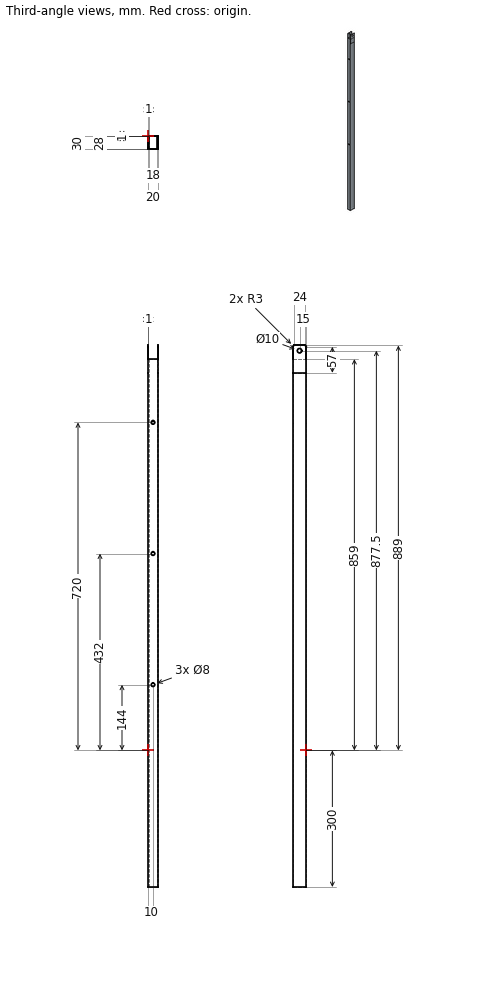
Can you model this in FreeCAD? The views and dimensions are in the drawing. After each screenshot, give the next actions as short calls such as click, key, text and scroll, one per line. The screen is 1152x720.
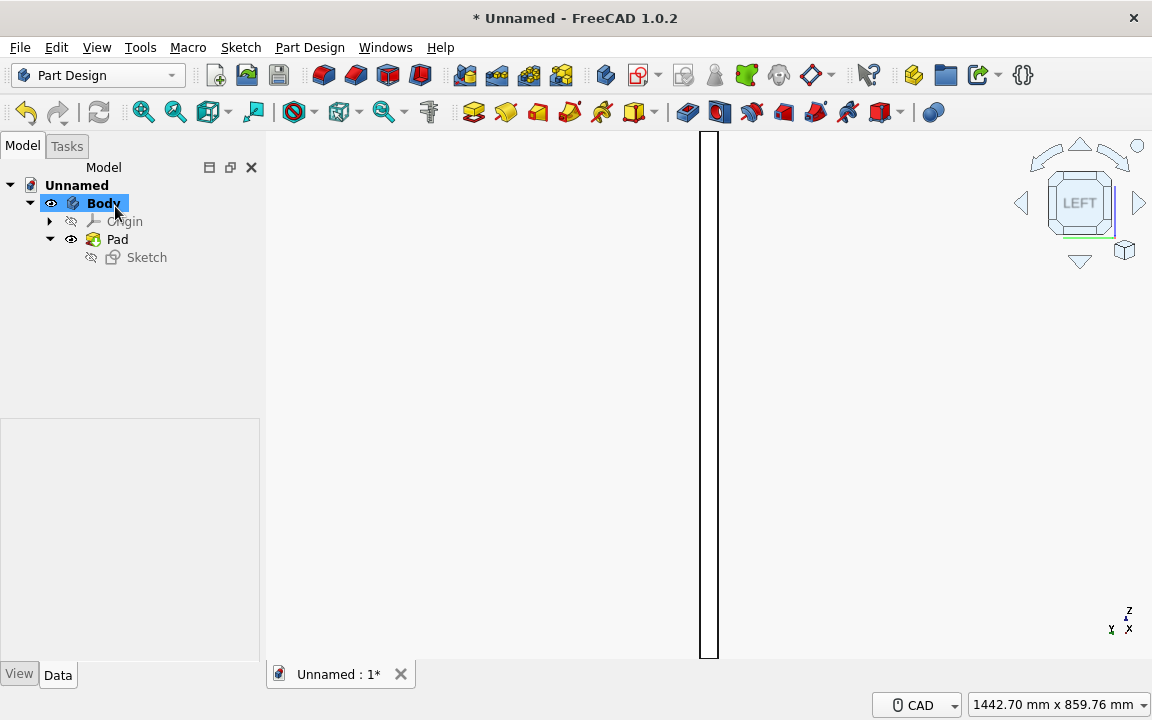
key(v)
key(f)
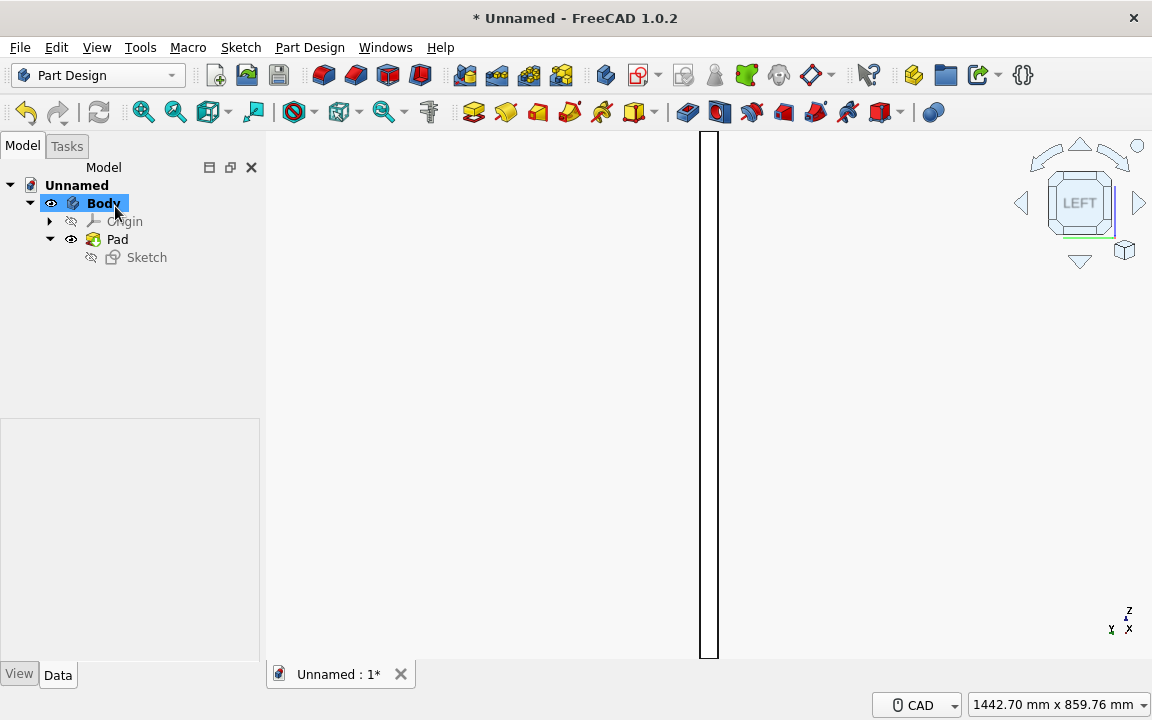
click(709, 168)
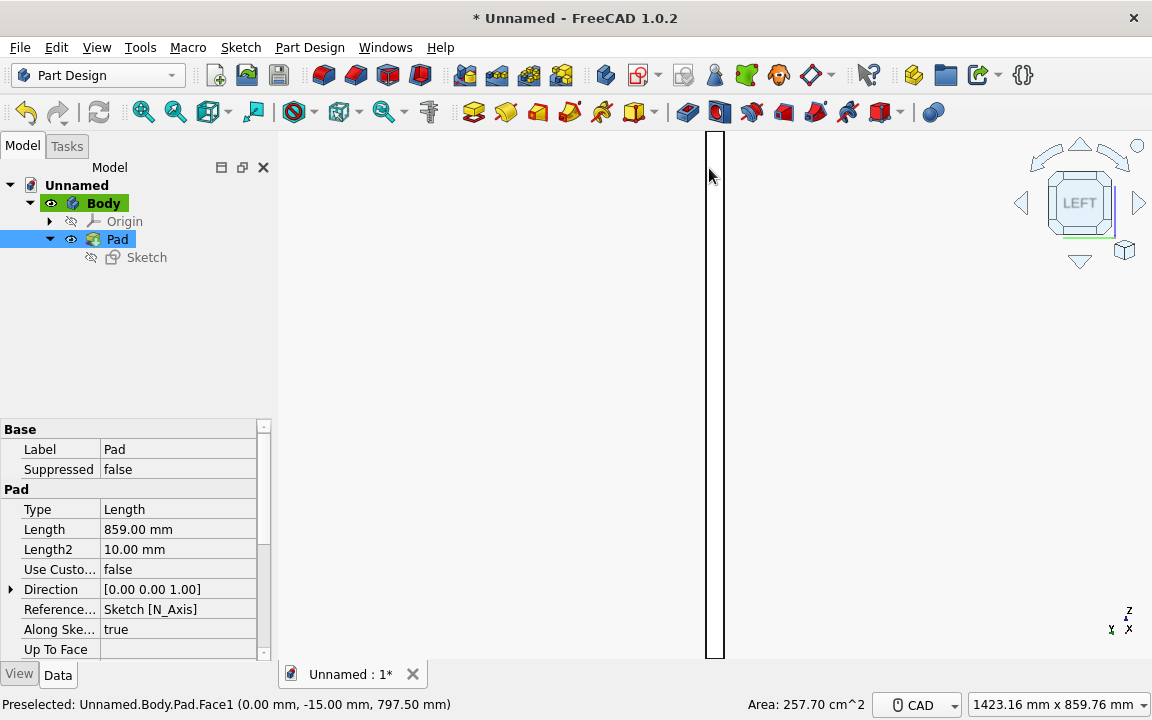
click(638, 76)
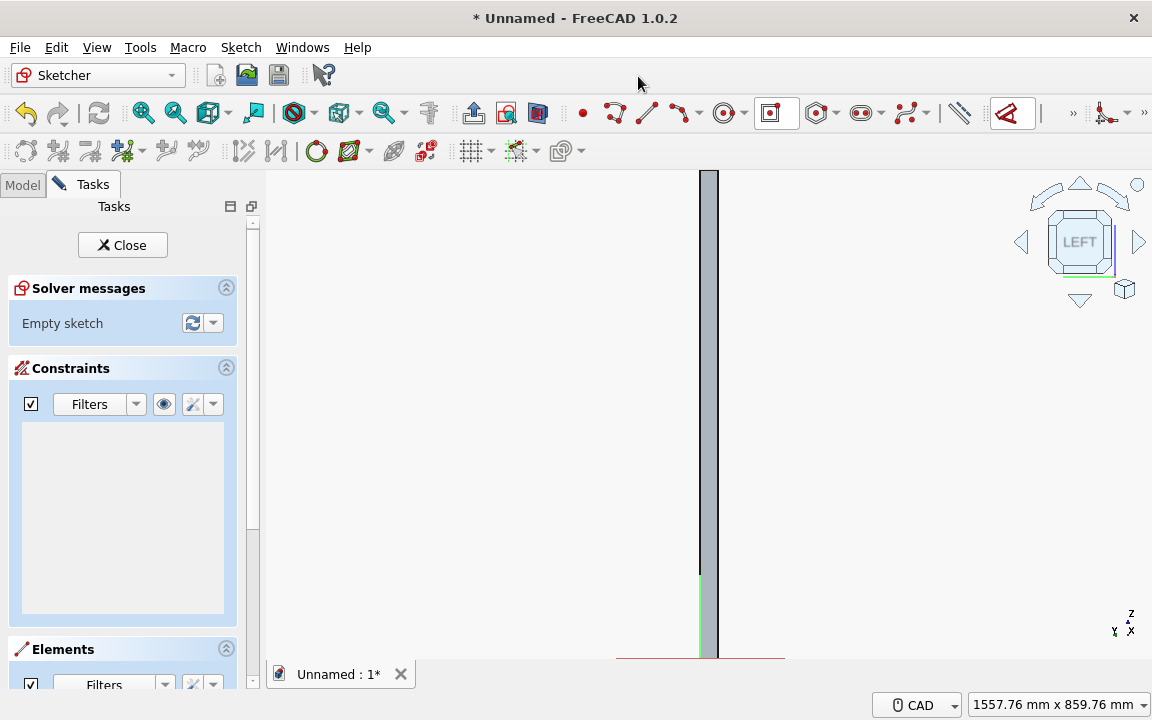
scroll(640, 414, down, 5)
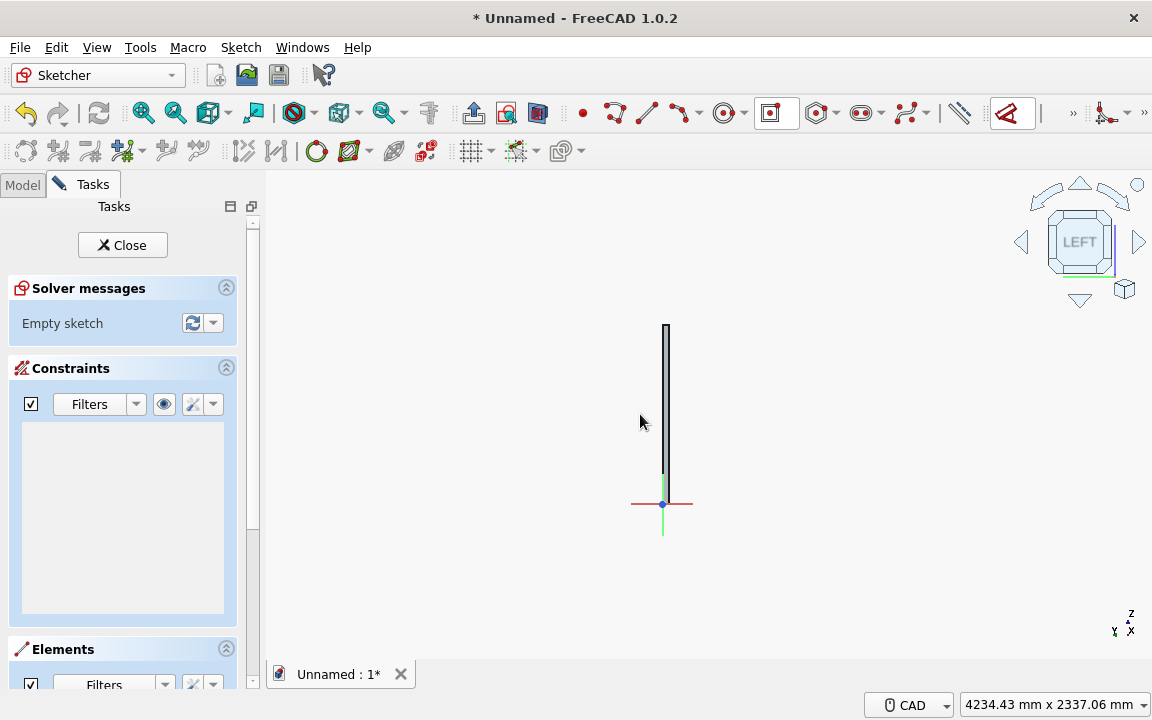
scroll(667, 320, up, 15)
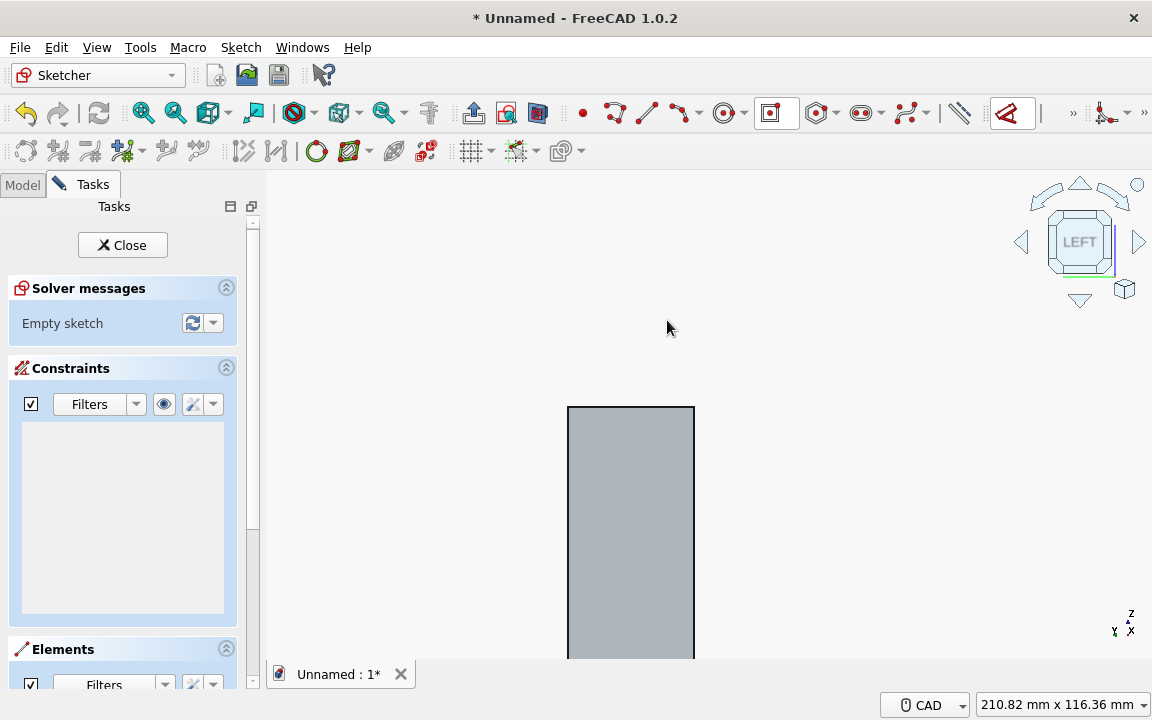
key(g)
key(l)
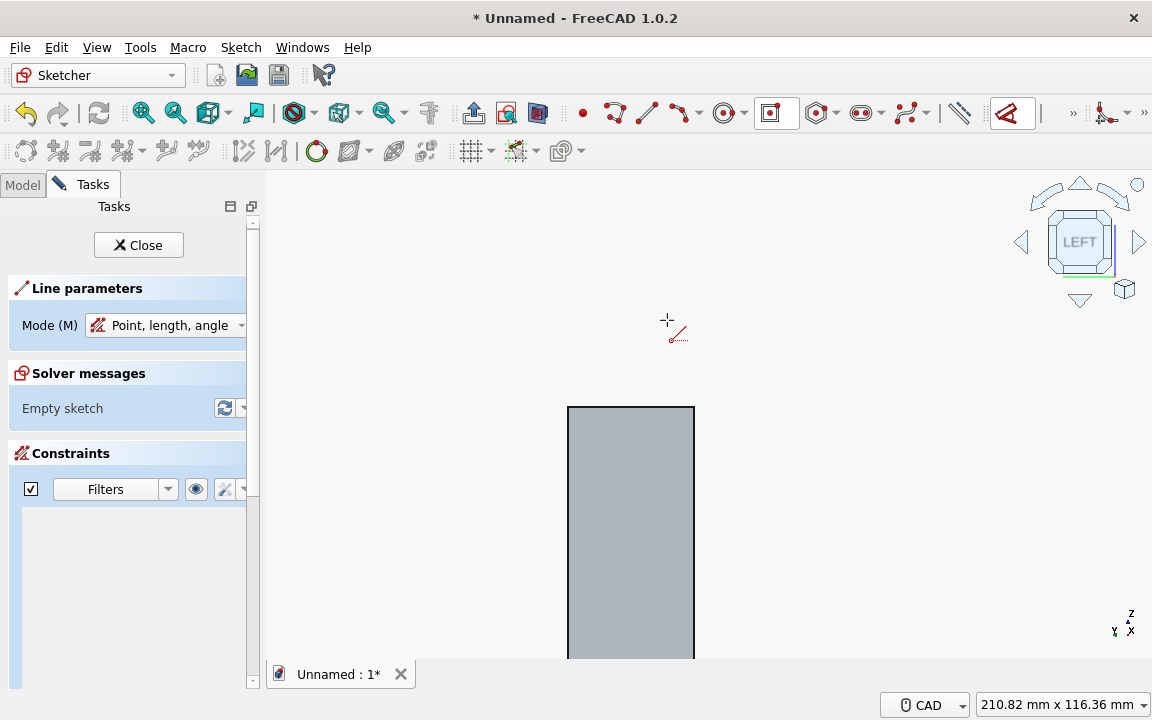
click(682, 281)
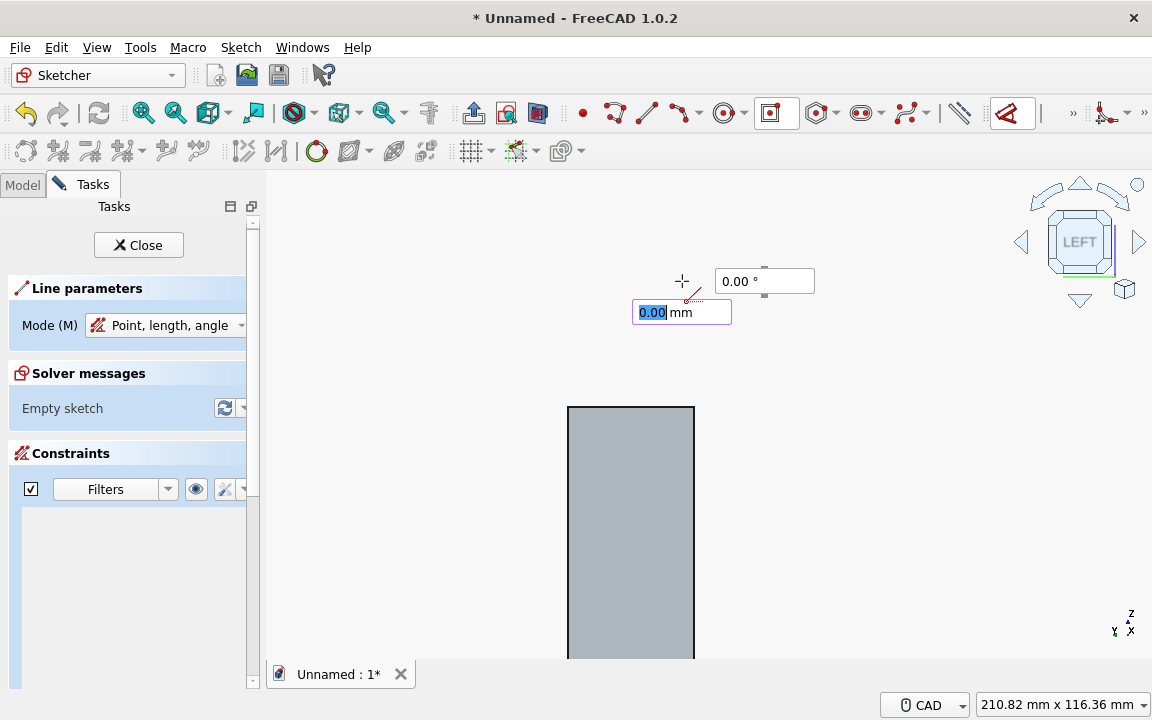
scroll(581, 281, up, 2)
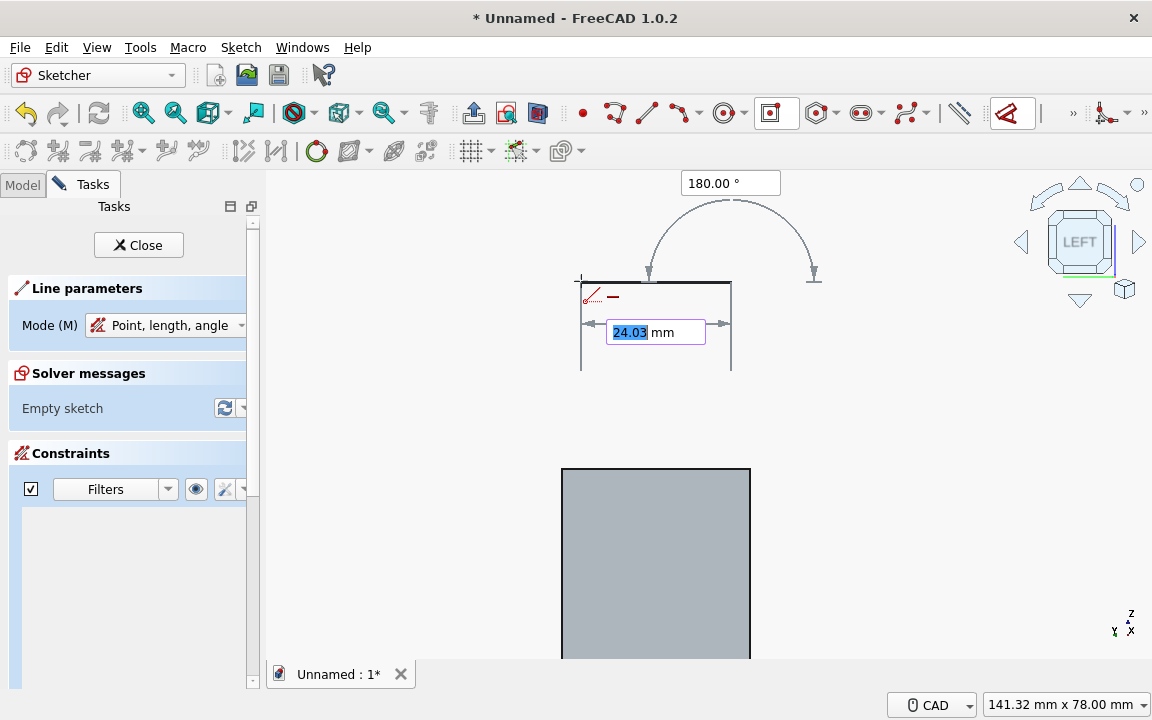
click(581, 281)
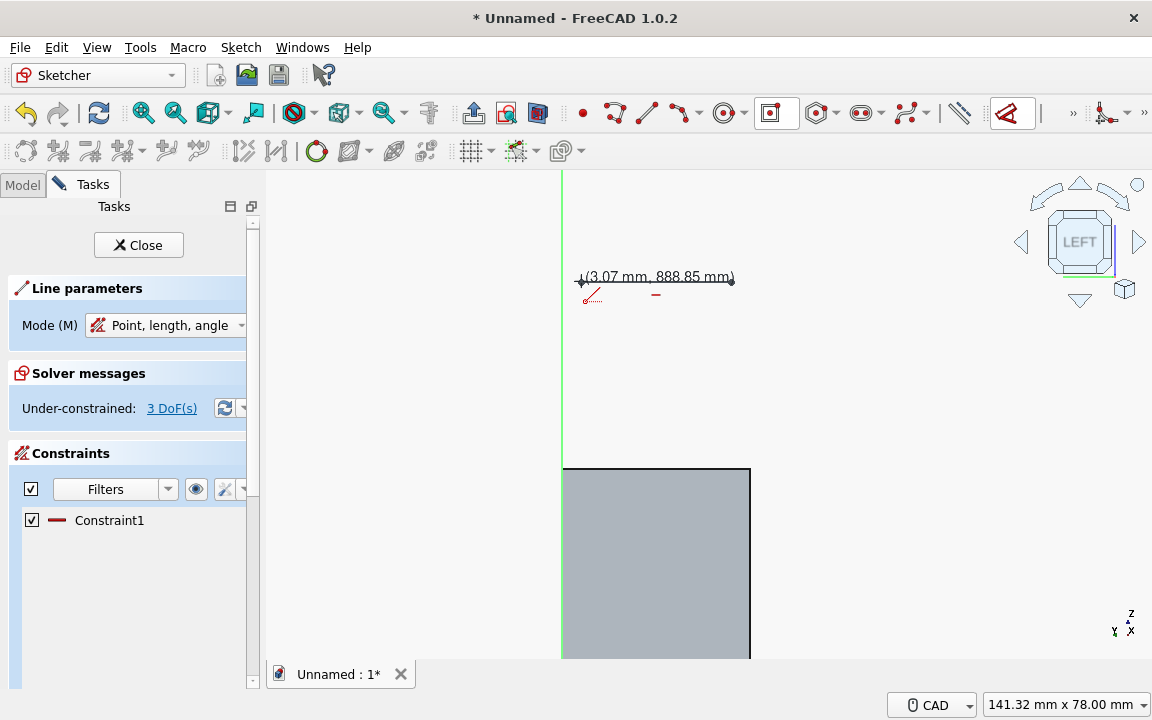
key(g)
key(m)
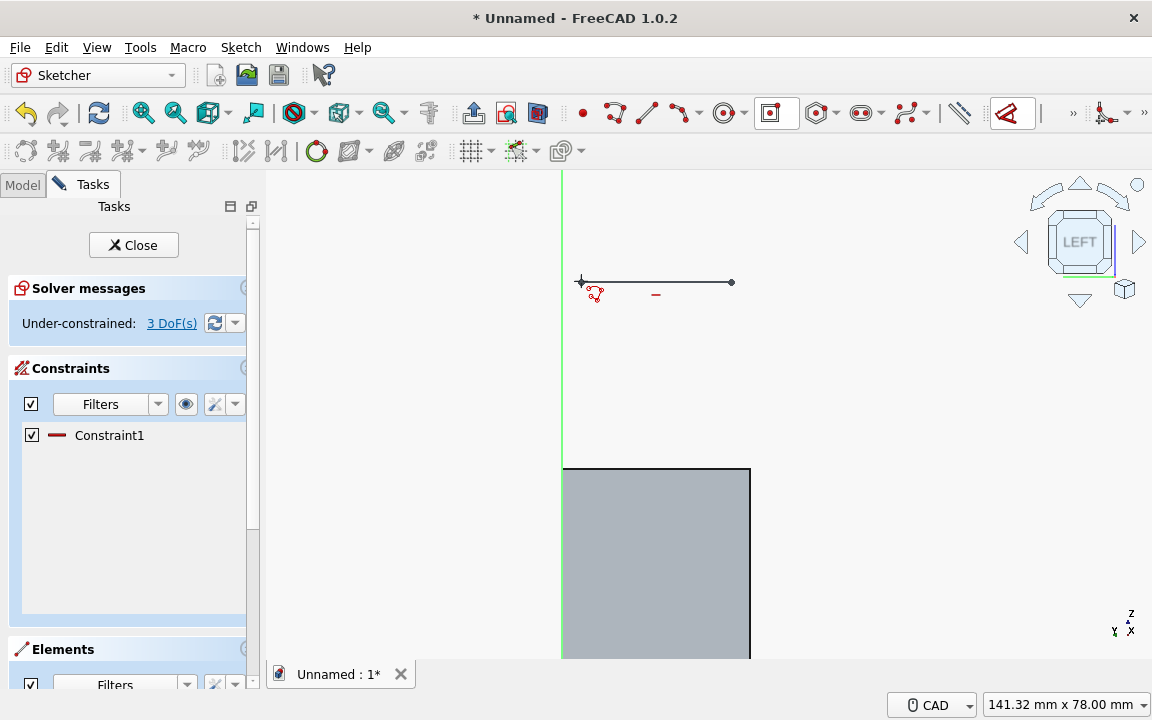
click(562, 300)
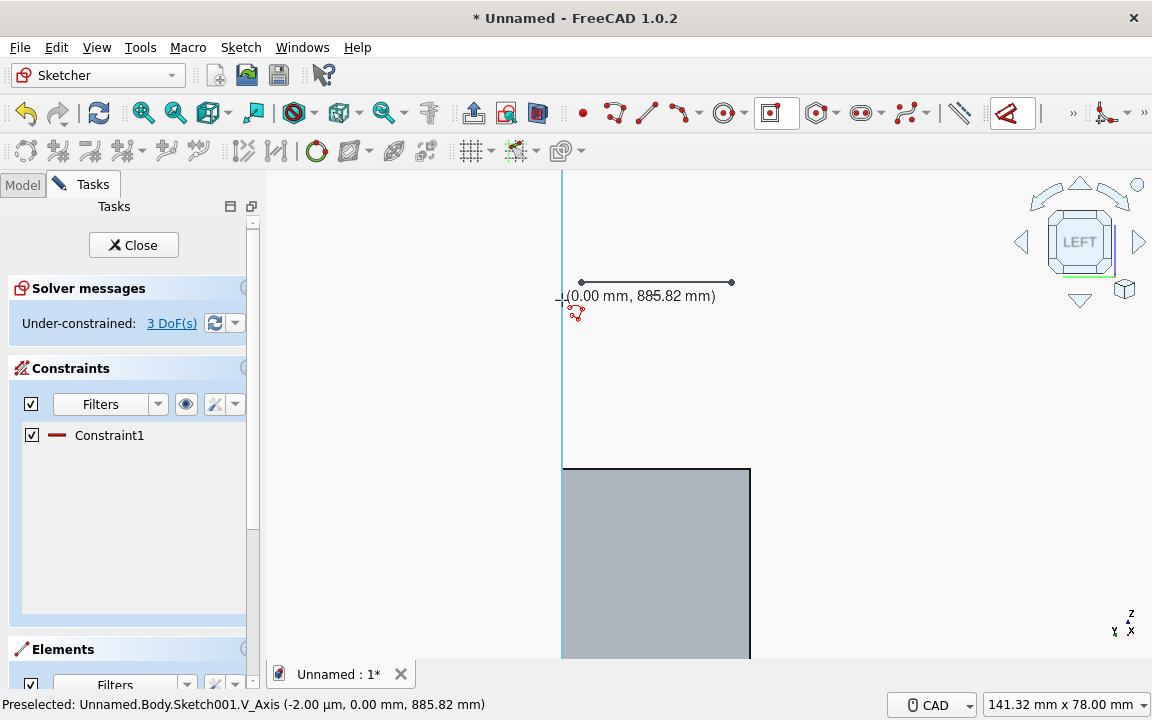
scroll(571, 198, down, 1)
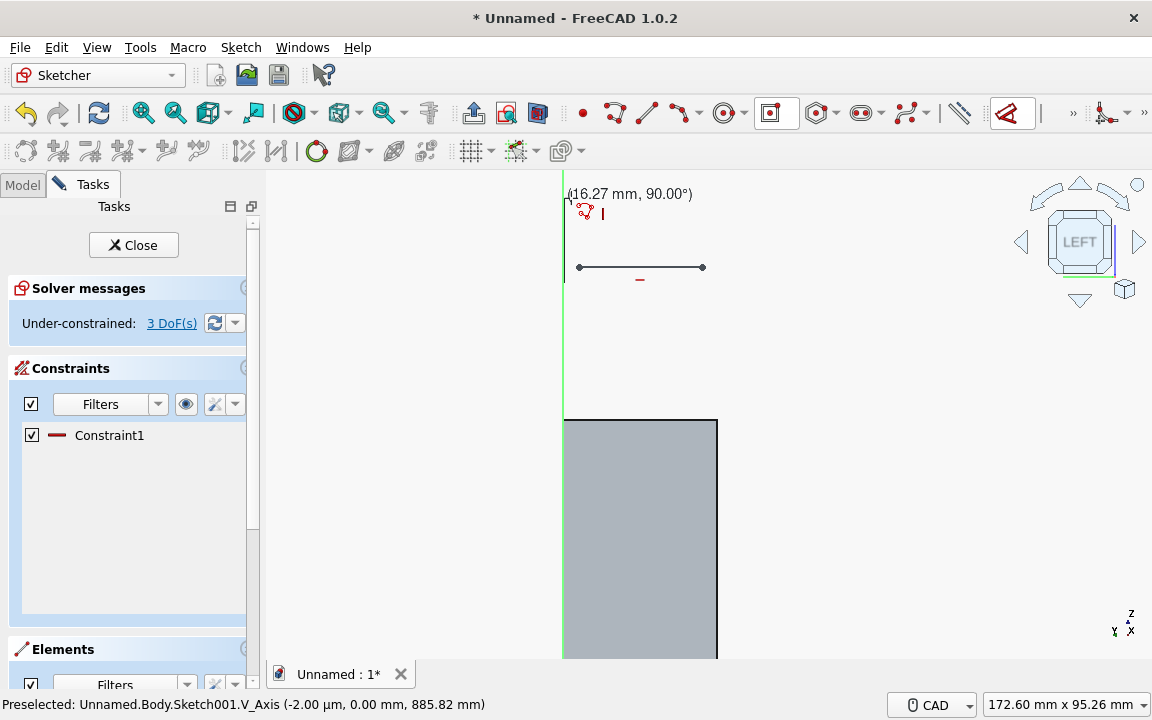
click(572, 574)
click(717, 574)
click(717, 281)
right_click(717, 281)